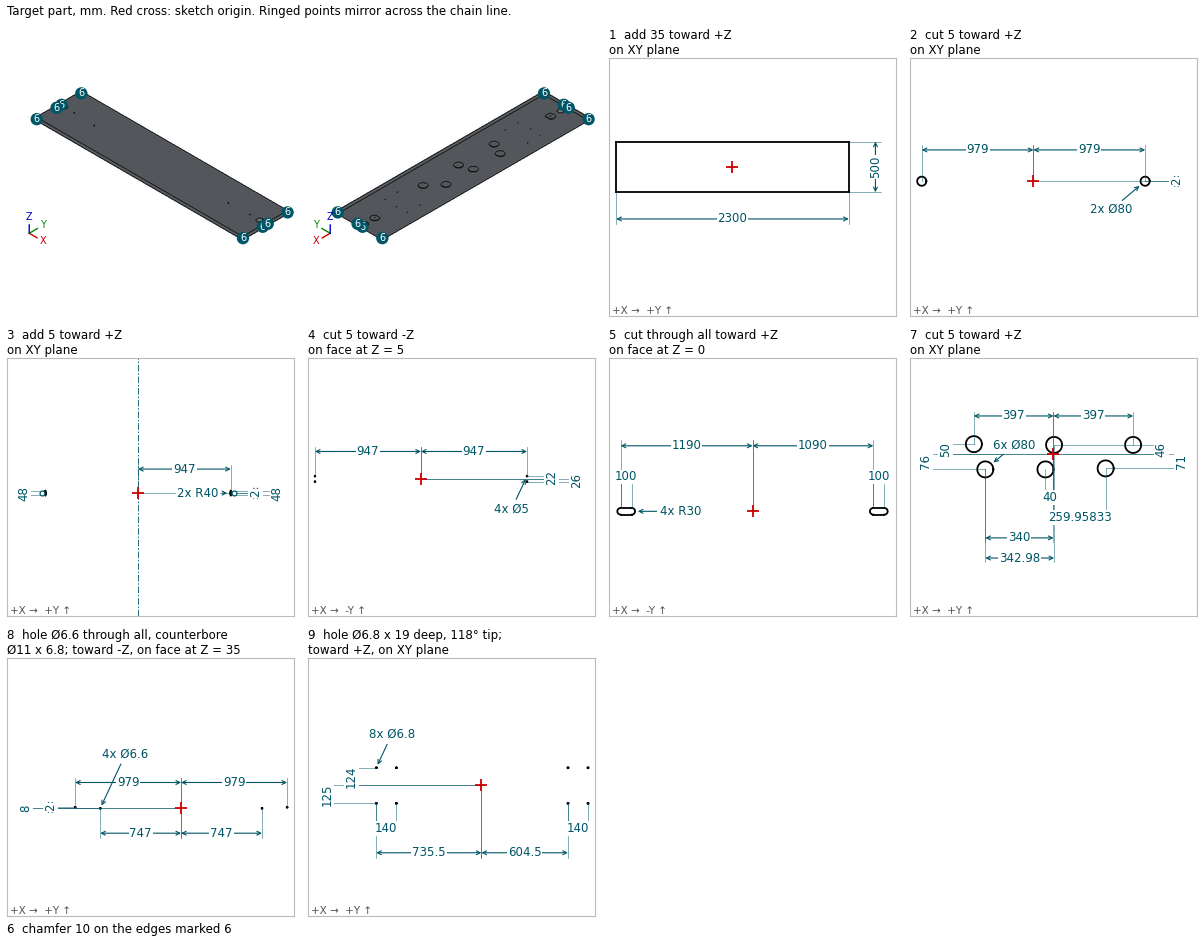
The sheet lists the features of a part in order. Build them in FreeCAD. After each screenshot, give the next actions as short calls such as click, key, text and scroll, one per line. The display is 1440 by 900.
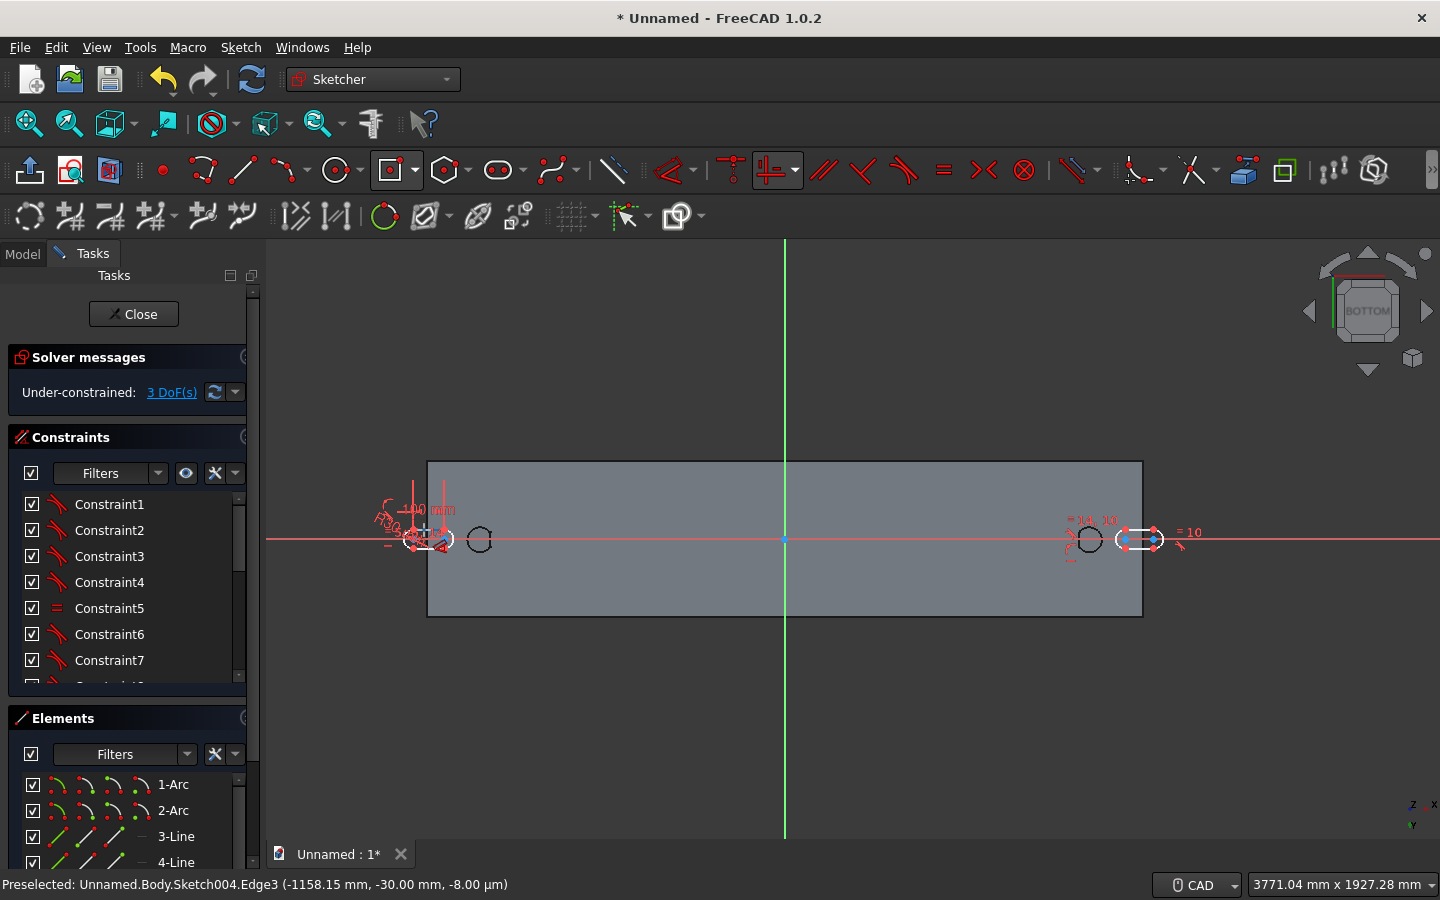
scroll(1134, 530, up, 3)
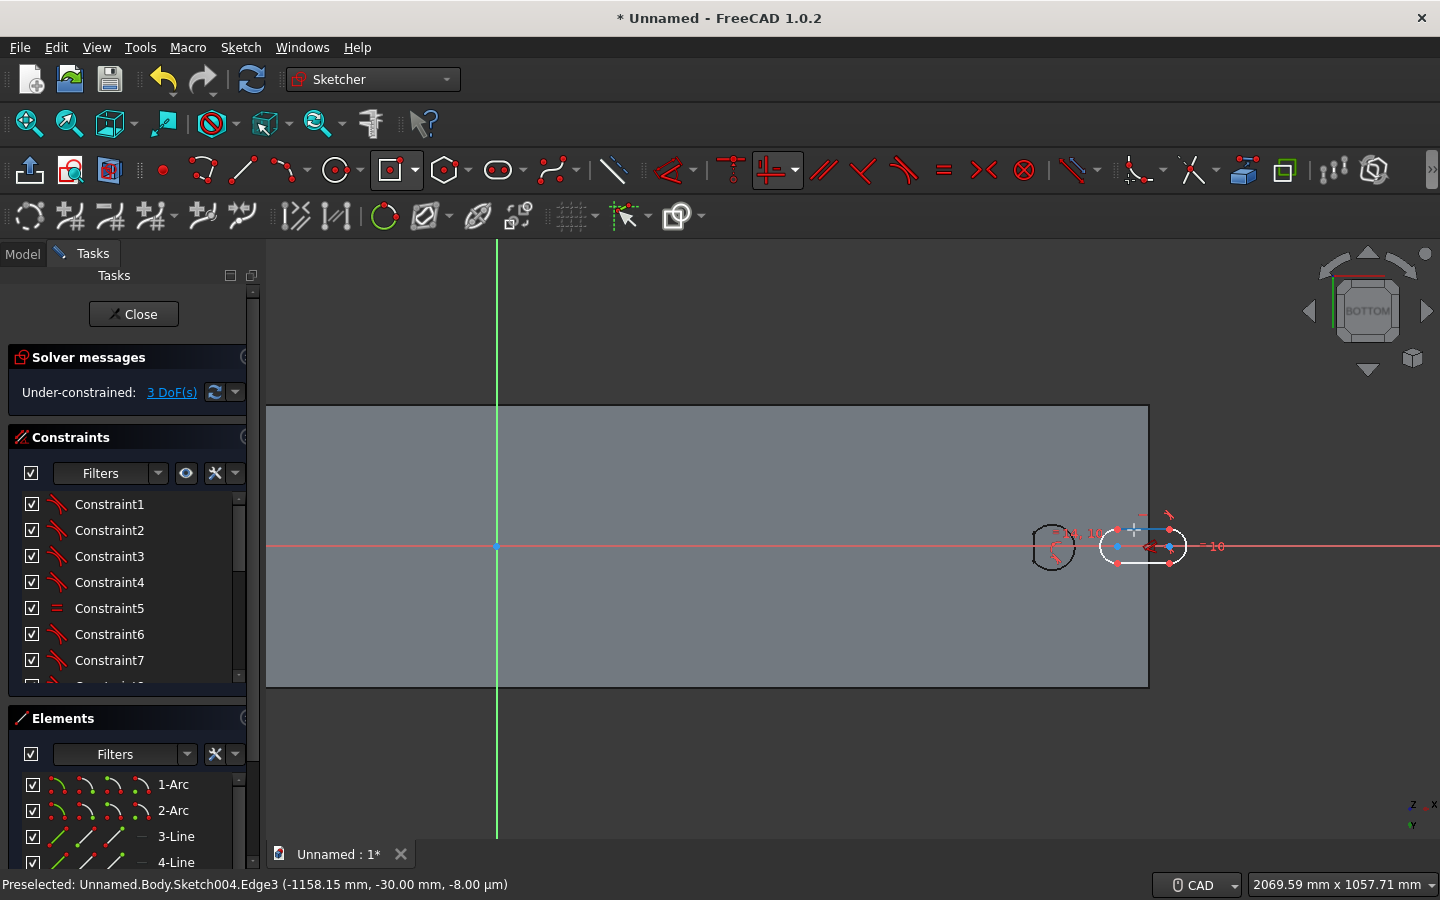
click(1133, 529)
click(1143, 495)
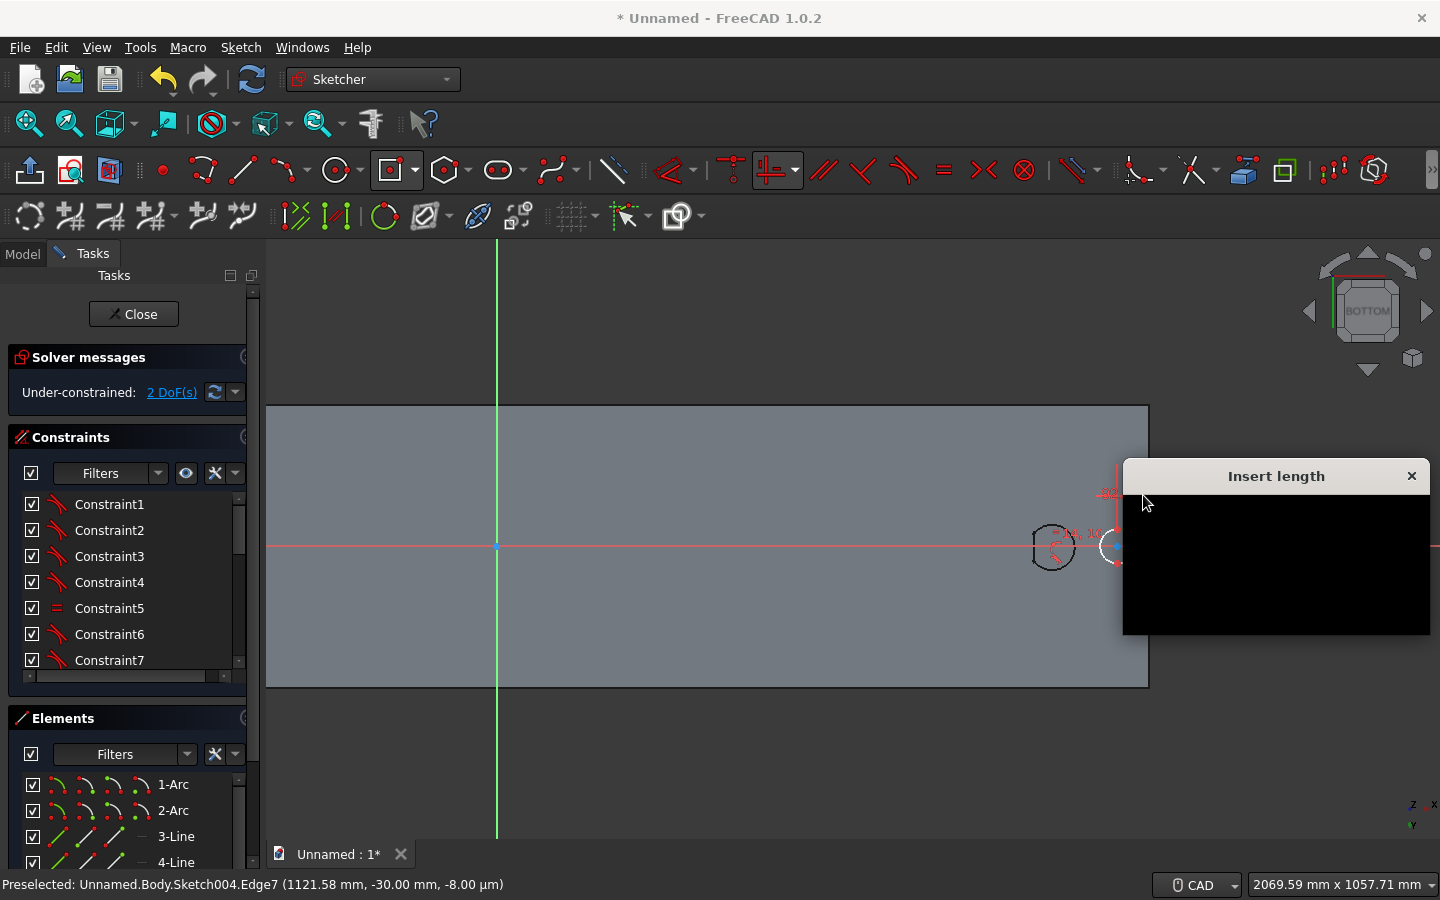
text(100)
key(Return)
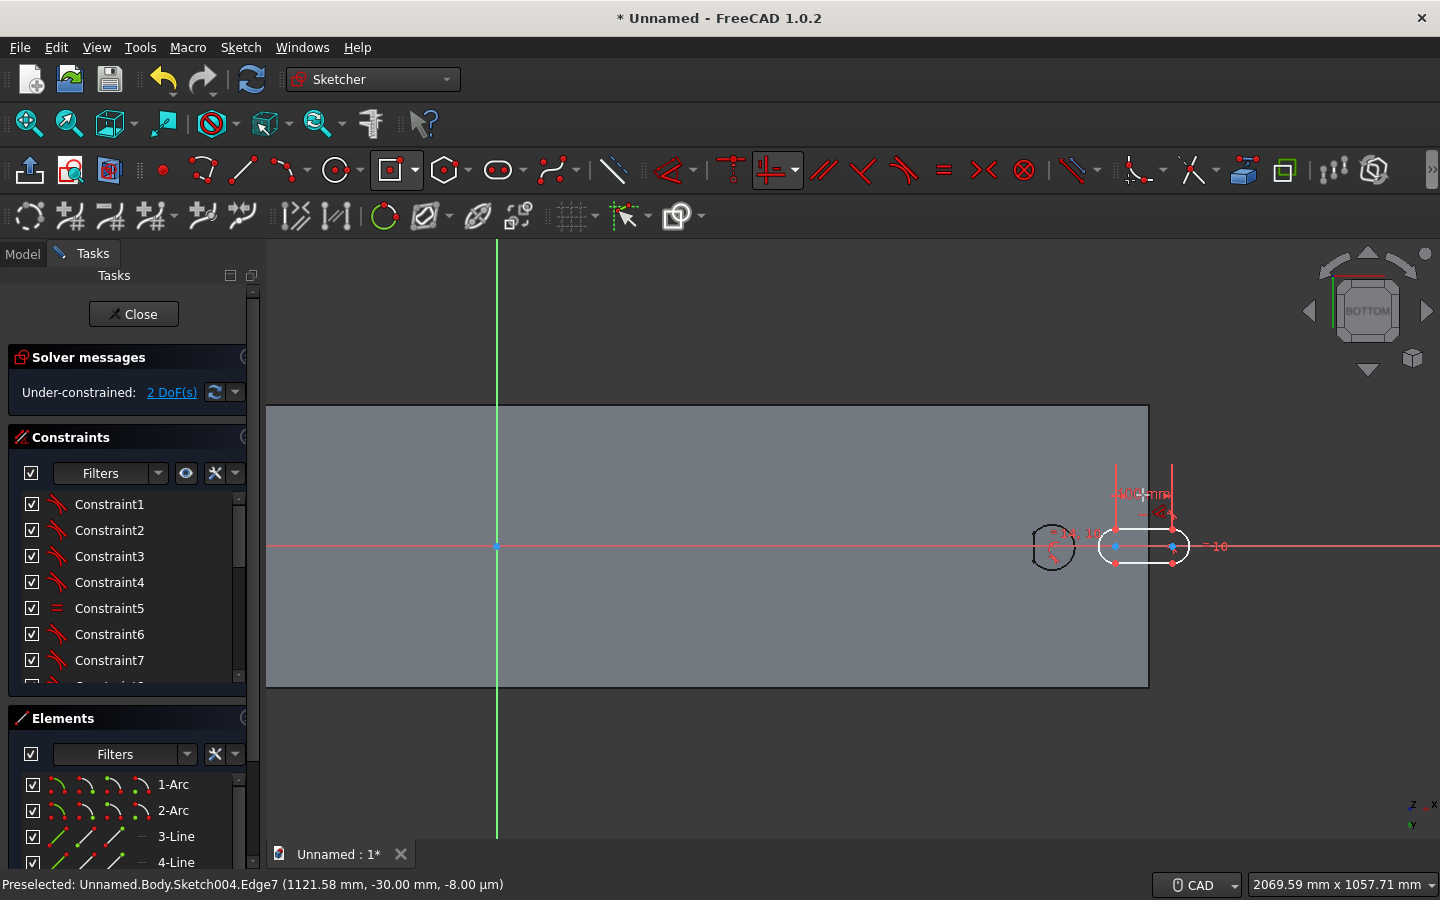
scroll(1134, 530, down, 3)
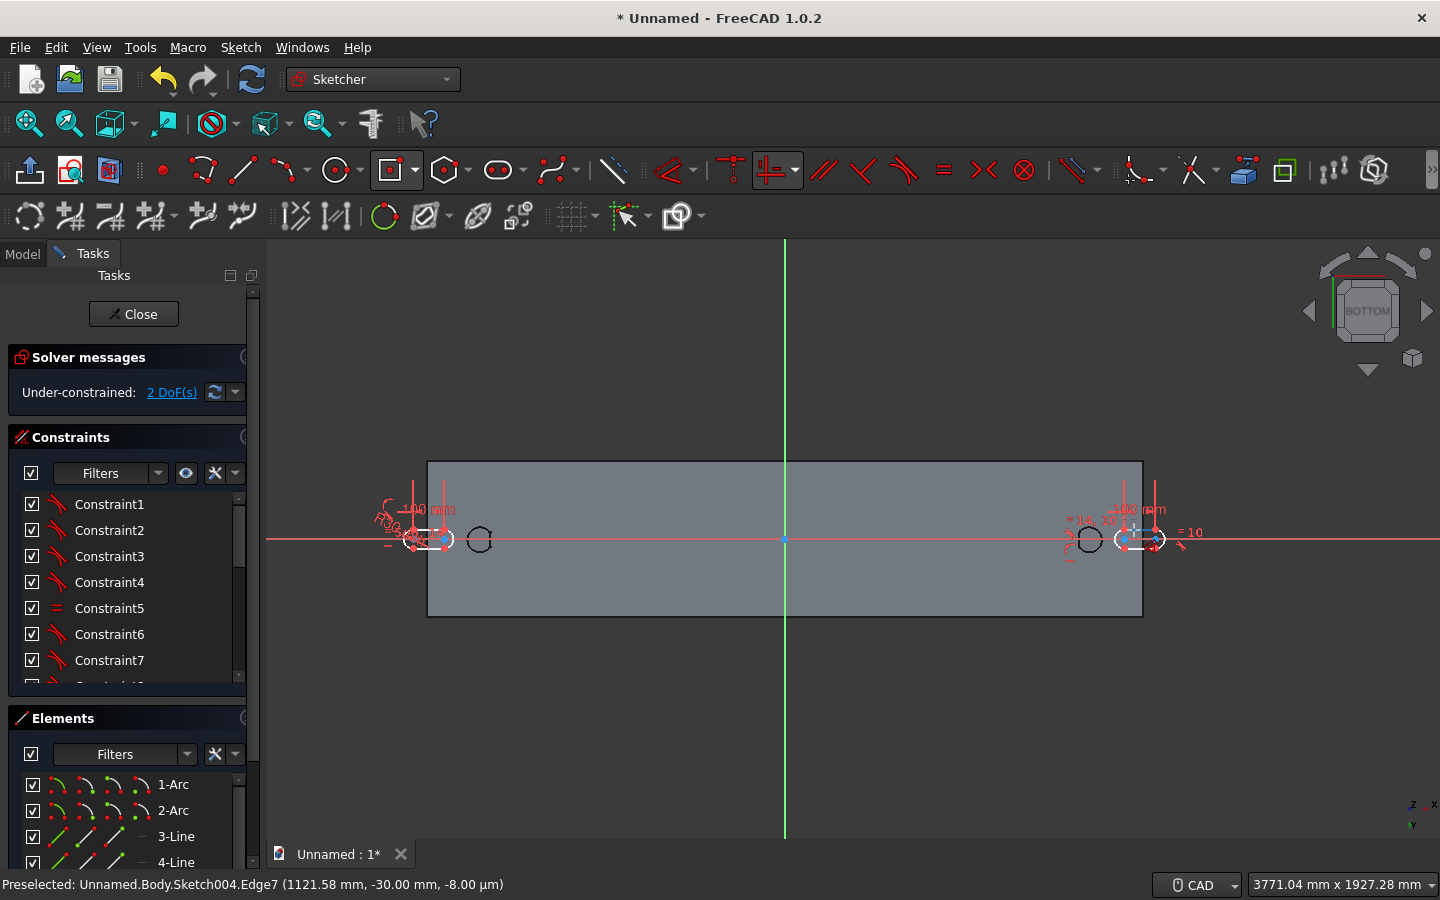
scroll(413, 530, up, 2)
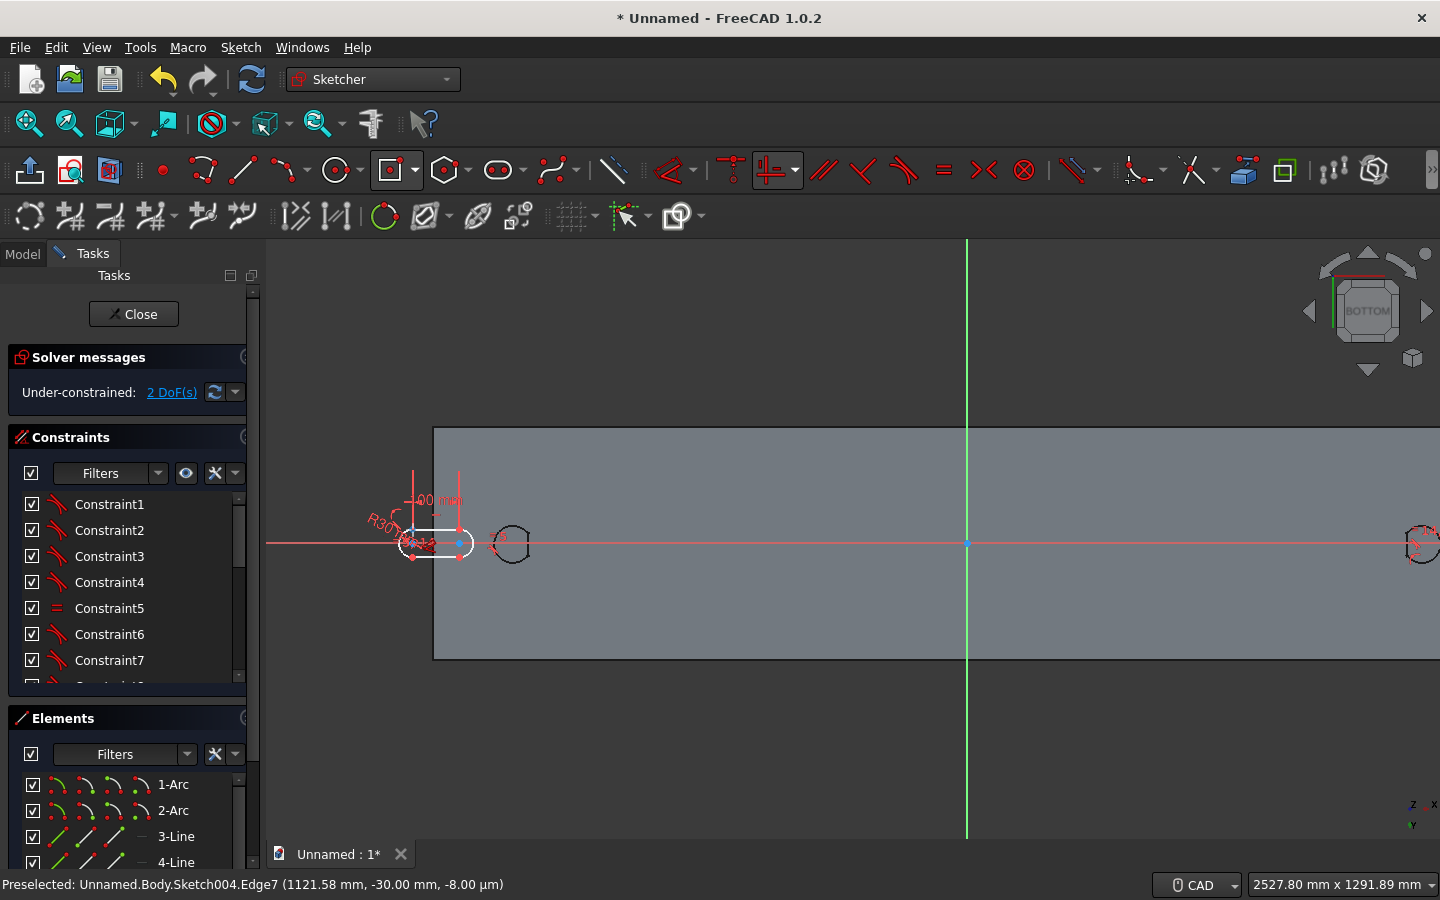
click(413, 530)
click(690, 496)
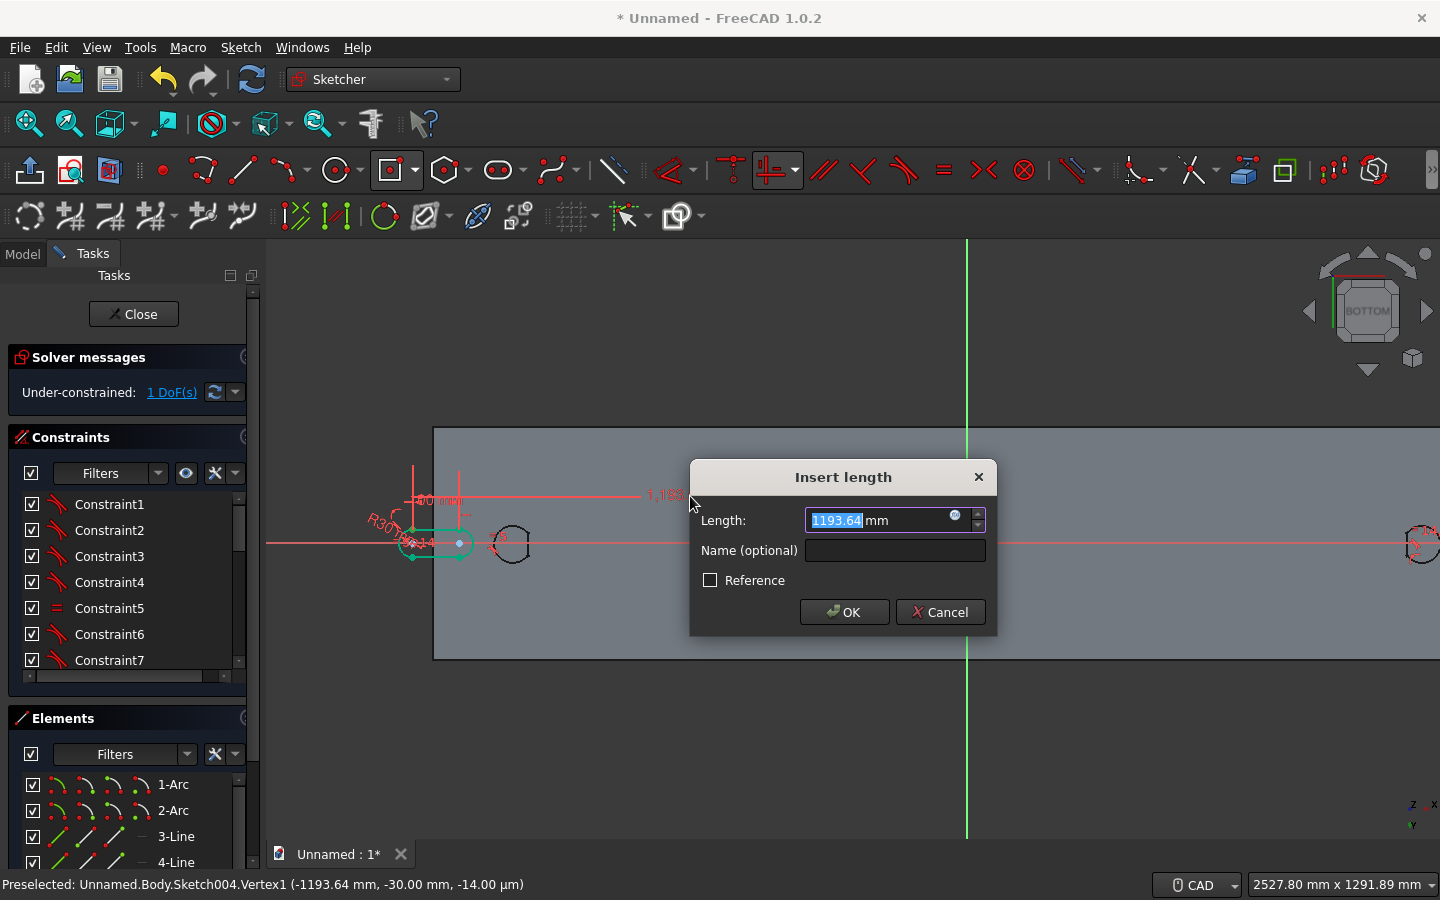
text(1190)
key(Return)